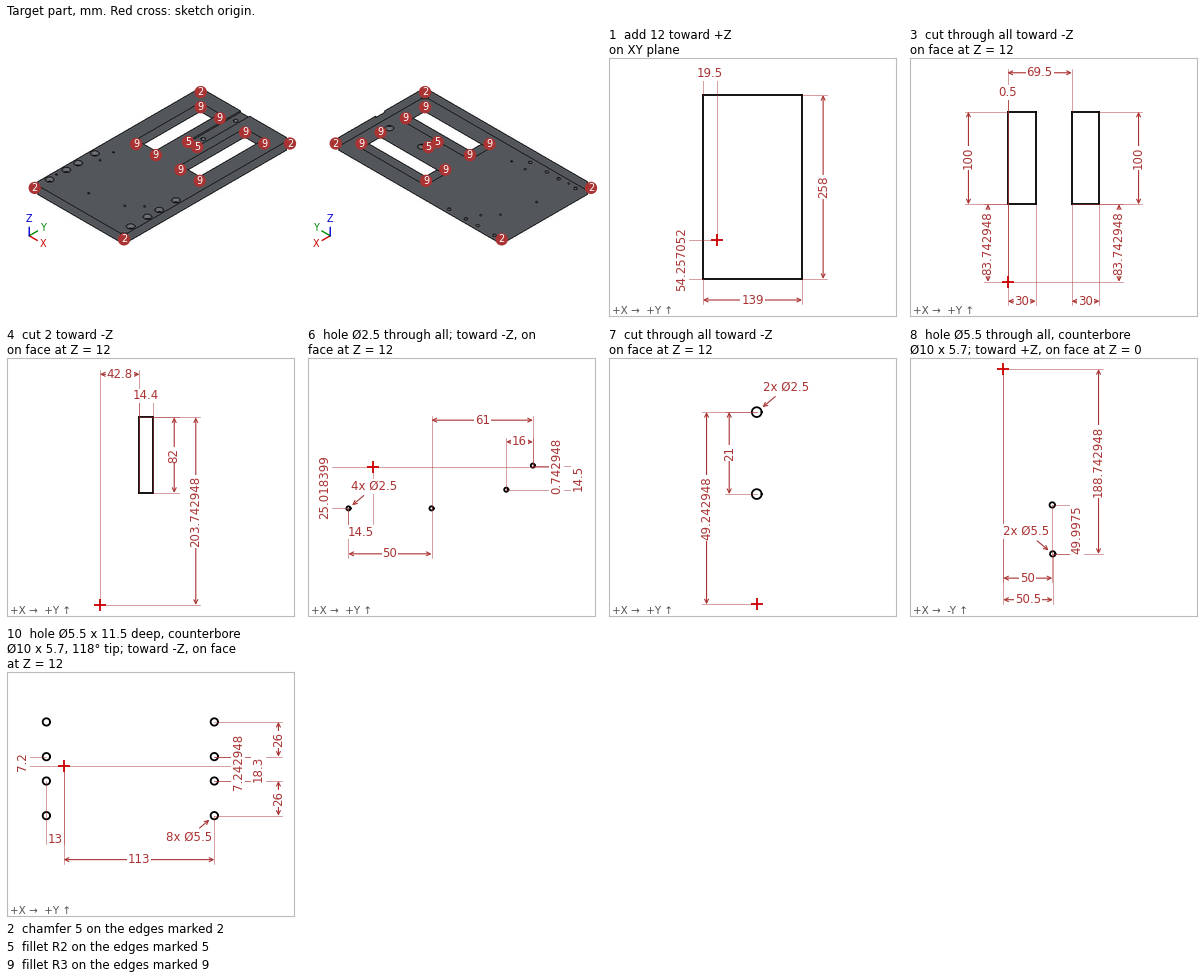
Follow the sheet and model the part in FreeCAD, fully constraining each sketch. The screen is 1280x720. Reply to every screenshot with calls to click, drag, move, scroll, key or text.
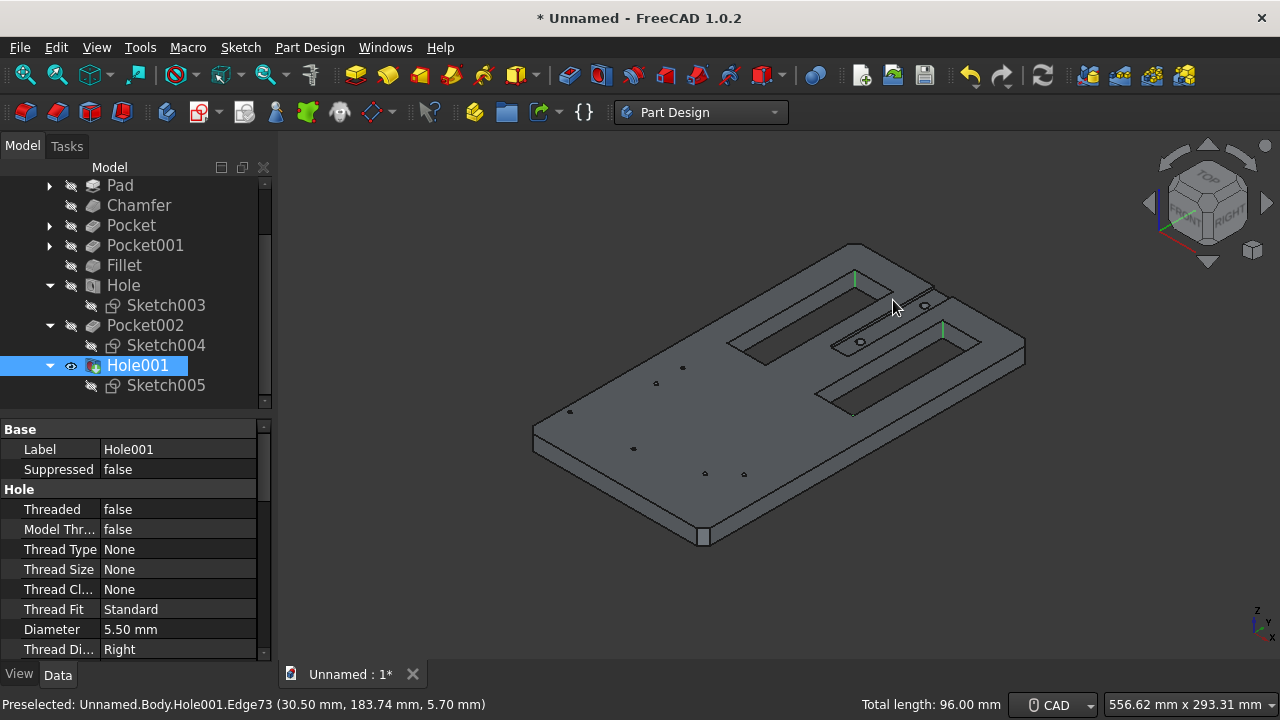
click(26, 112)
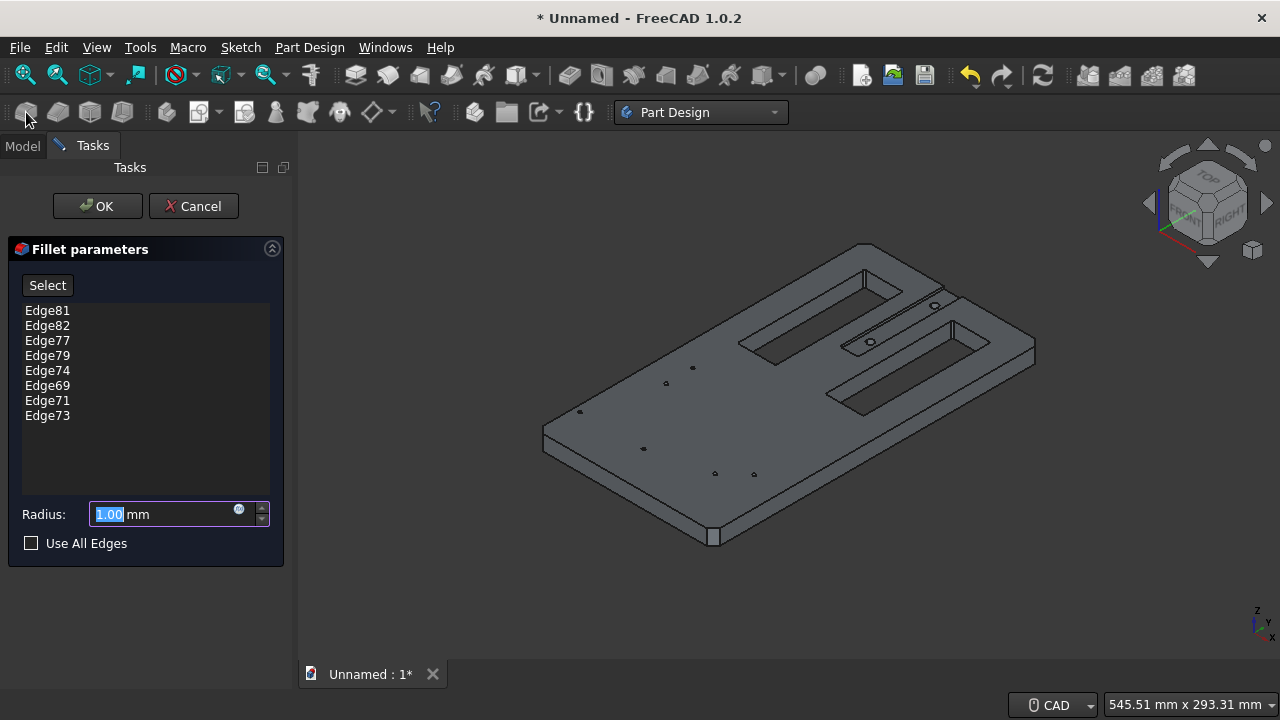
text(3)
key(Tab)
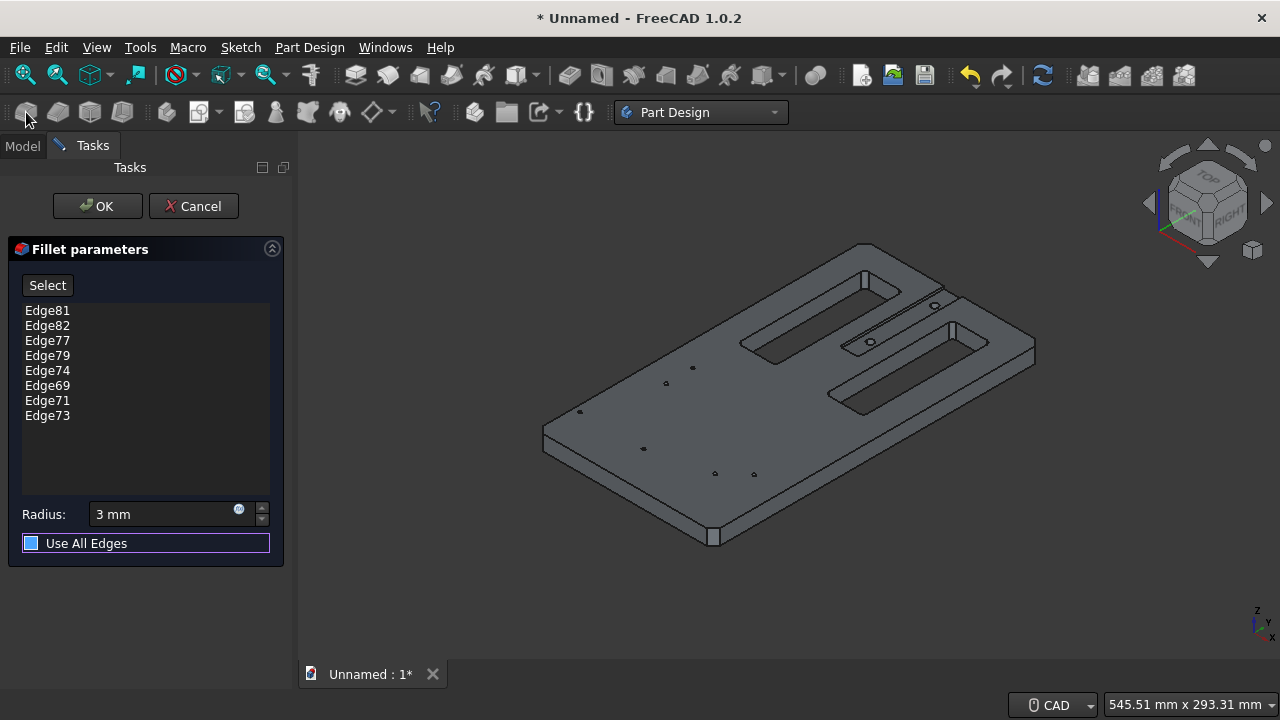
click(98, 206)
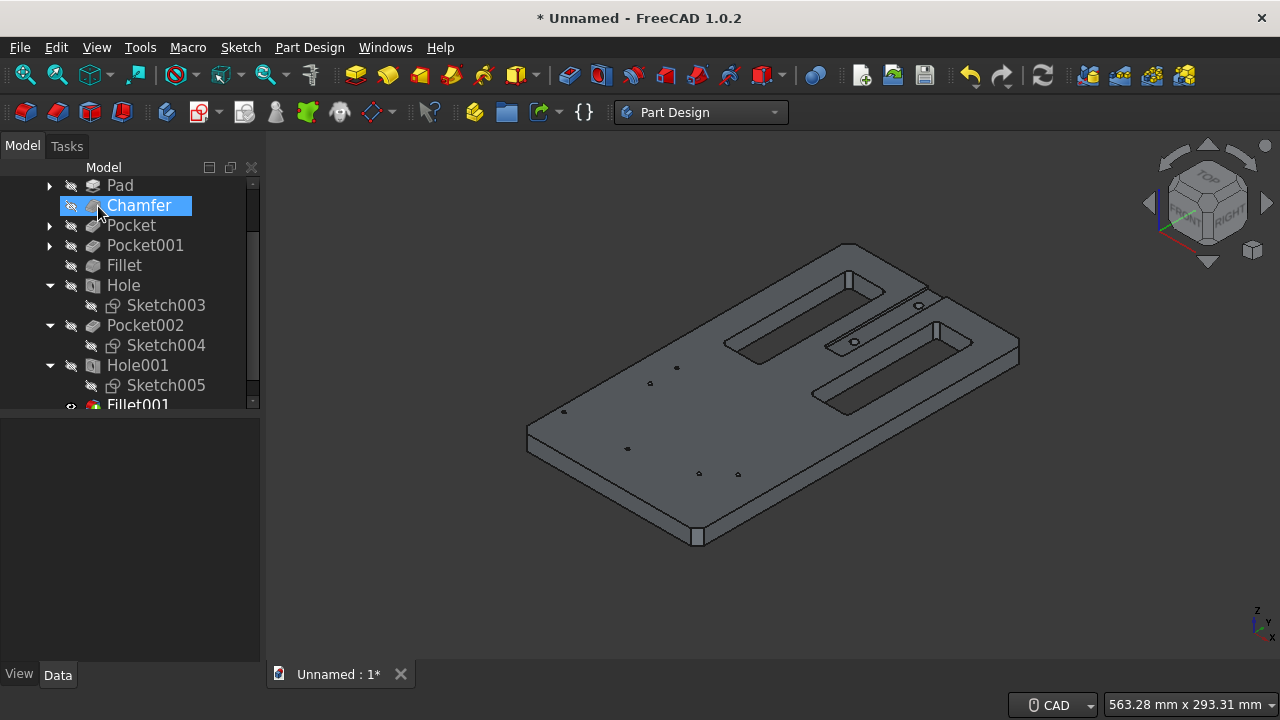
click(726, 412)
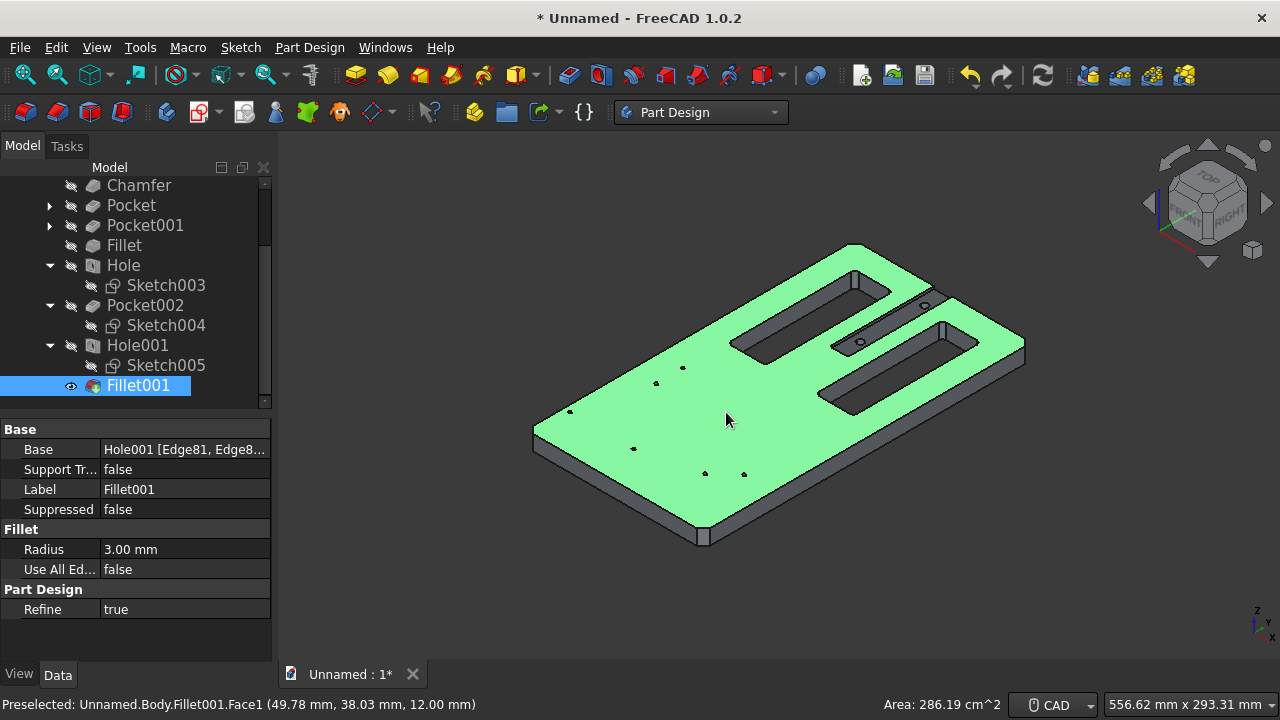
click(200, 112)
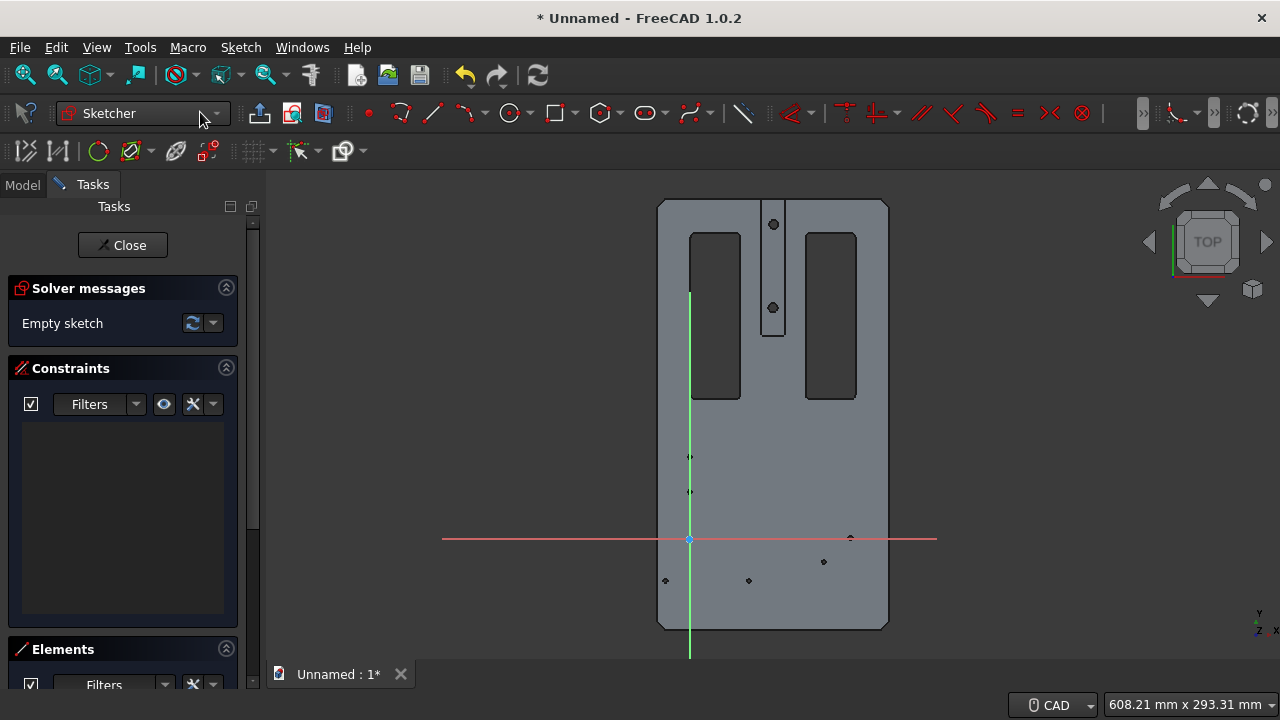
scroll(829, 631, up, 4)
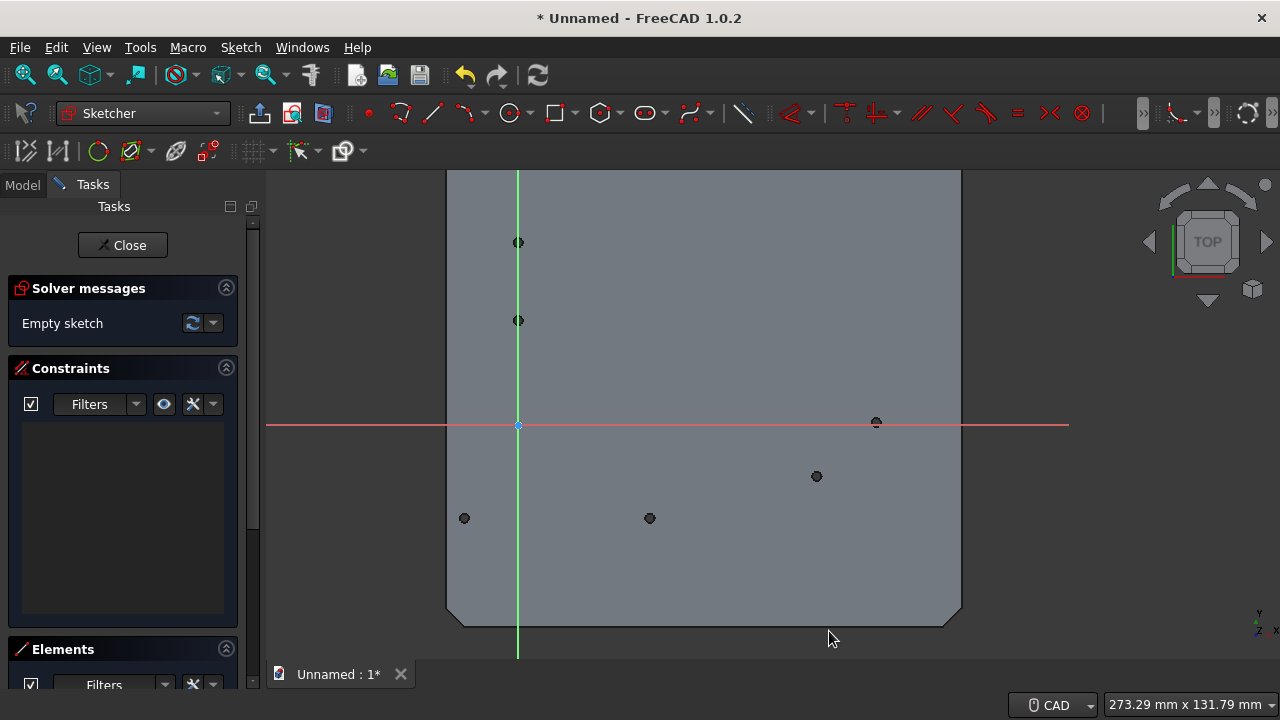
key(g)
key(c)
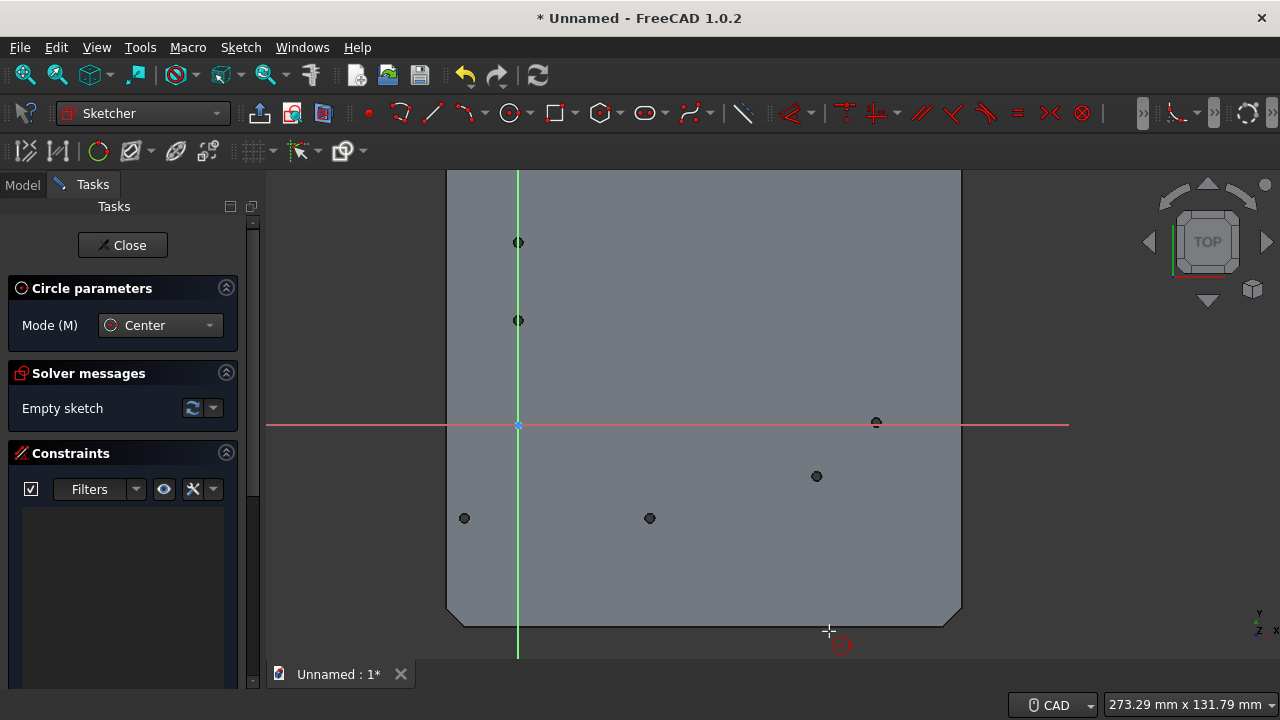
scroll(937, 563, up, 4)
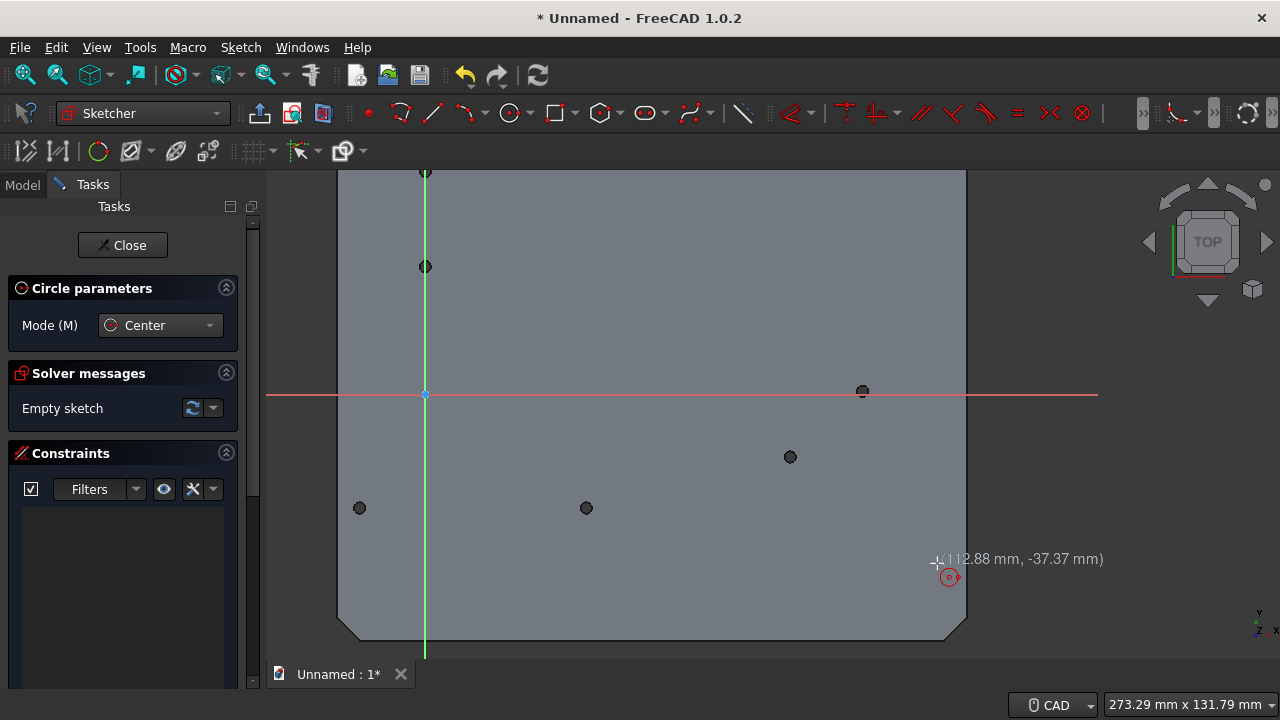
click(937, 562)
move(953, 546)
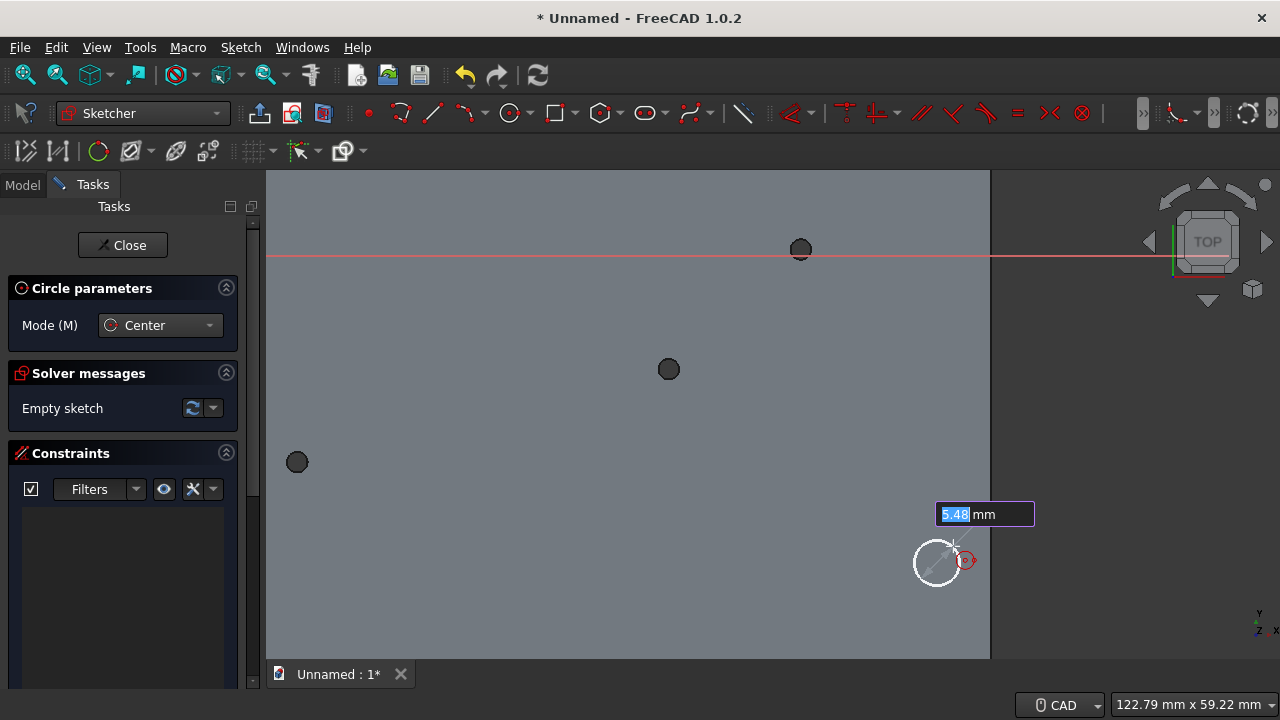
text(5.5)
key(Return)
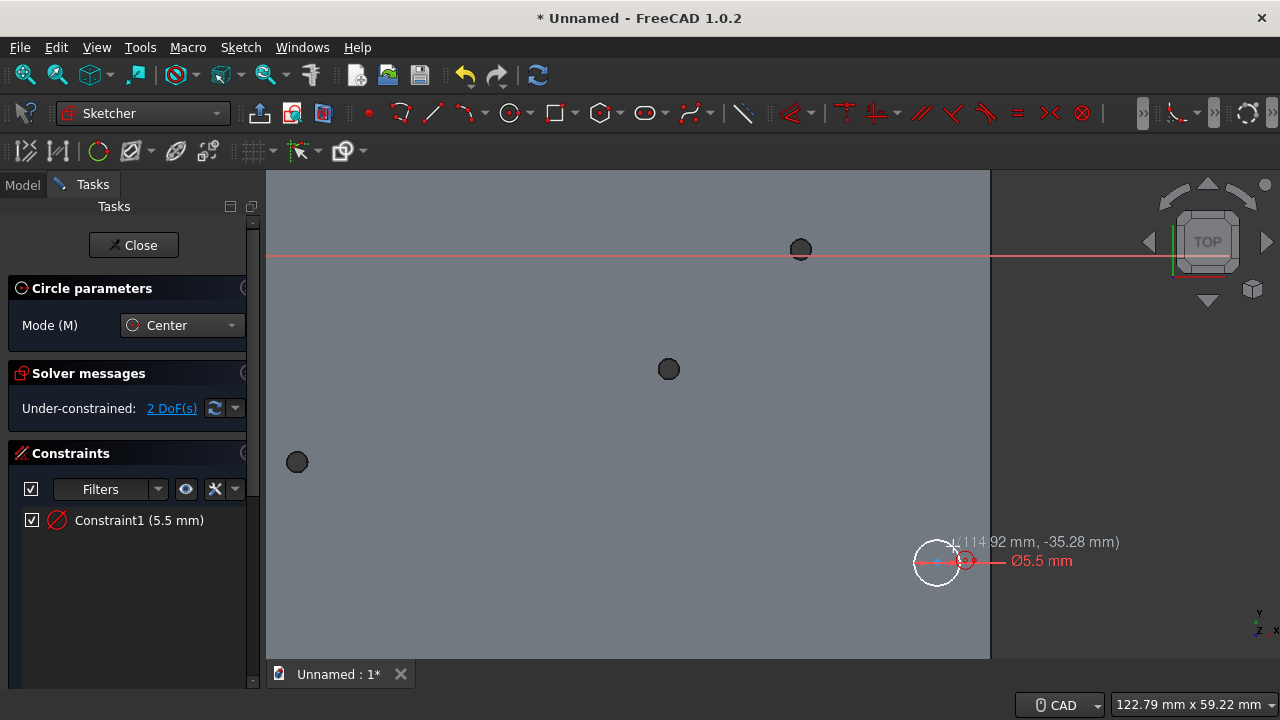
click(937, 347)
move(953, 331)